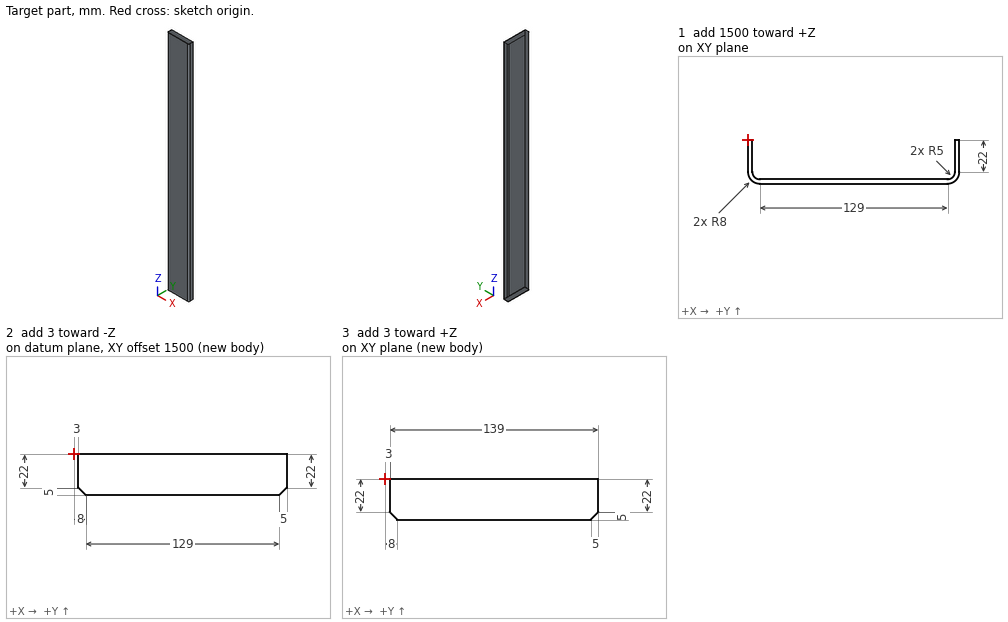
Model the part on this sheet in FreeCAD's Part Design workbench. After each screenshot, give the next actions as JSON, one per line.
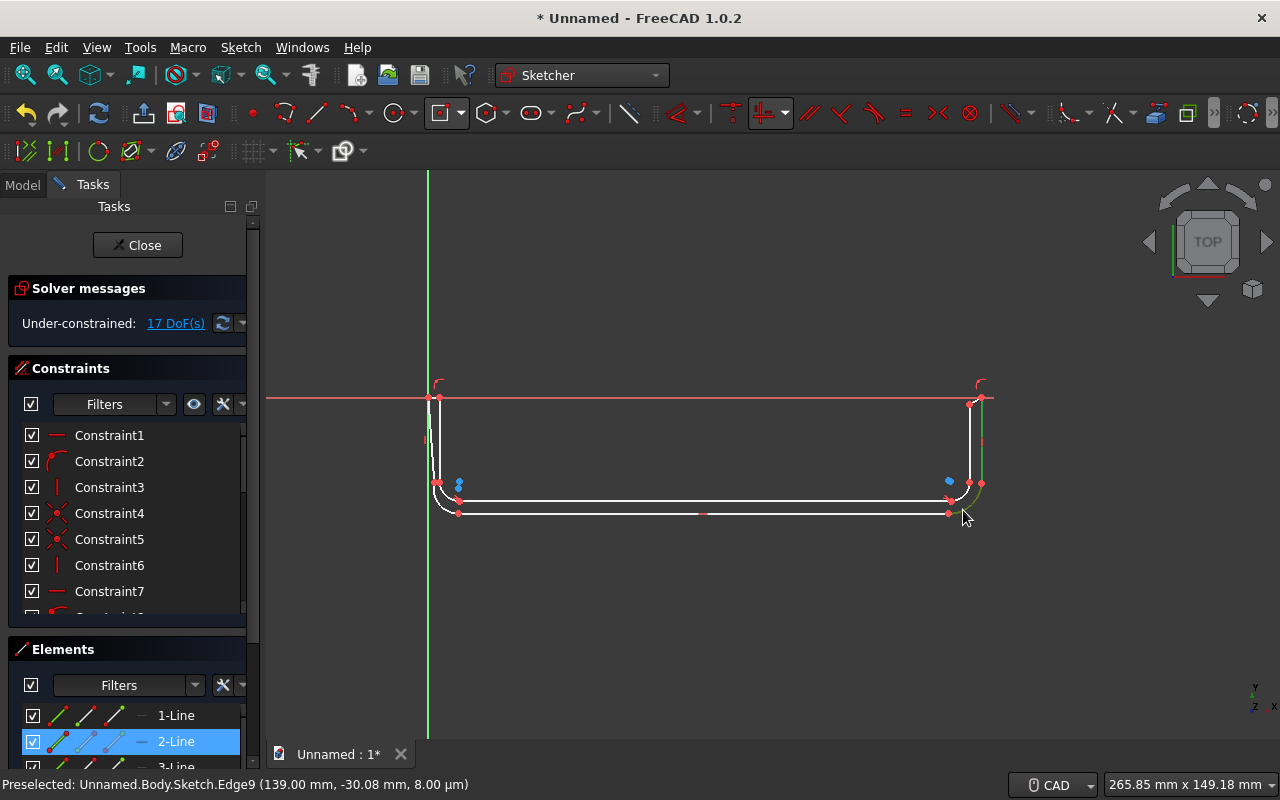
{"action": "key", "text": "t"}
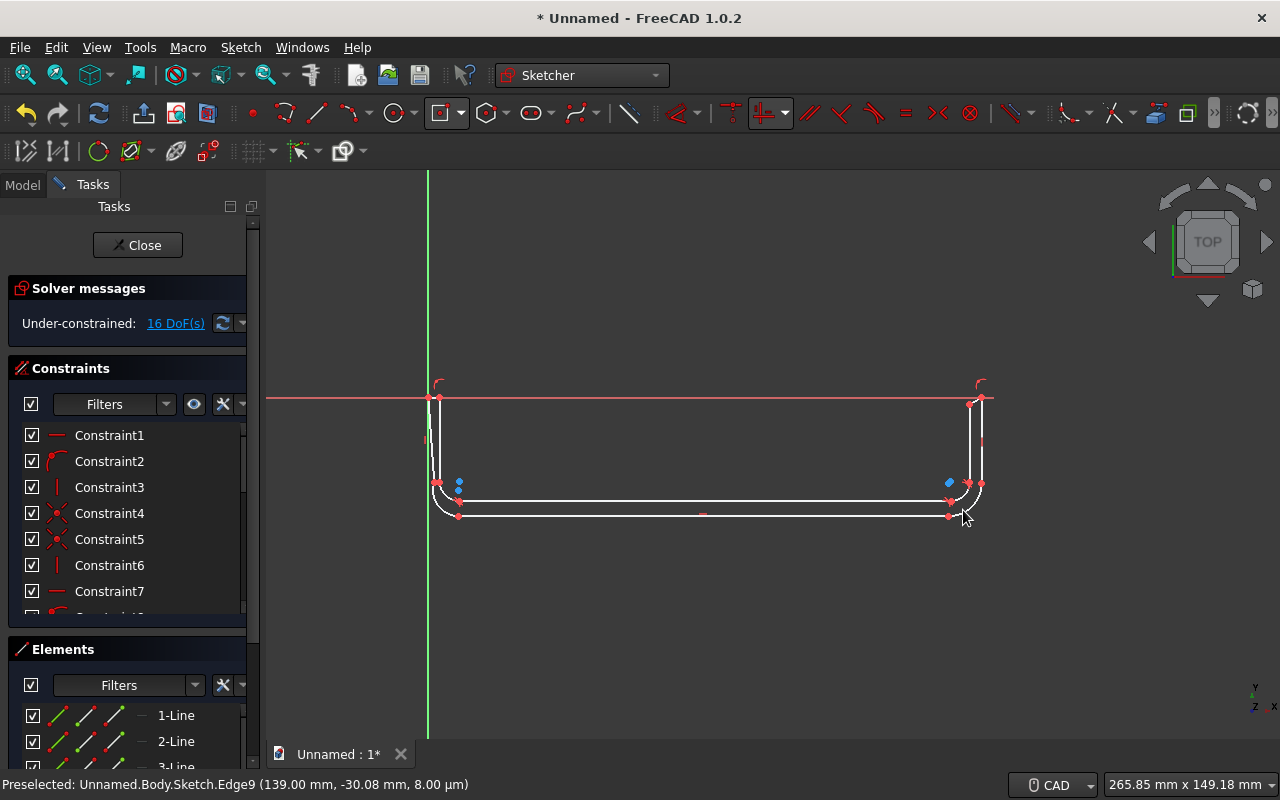
{"action": "left_click", "coordinate": [970, 428]}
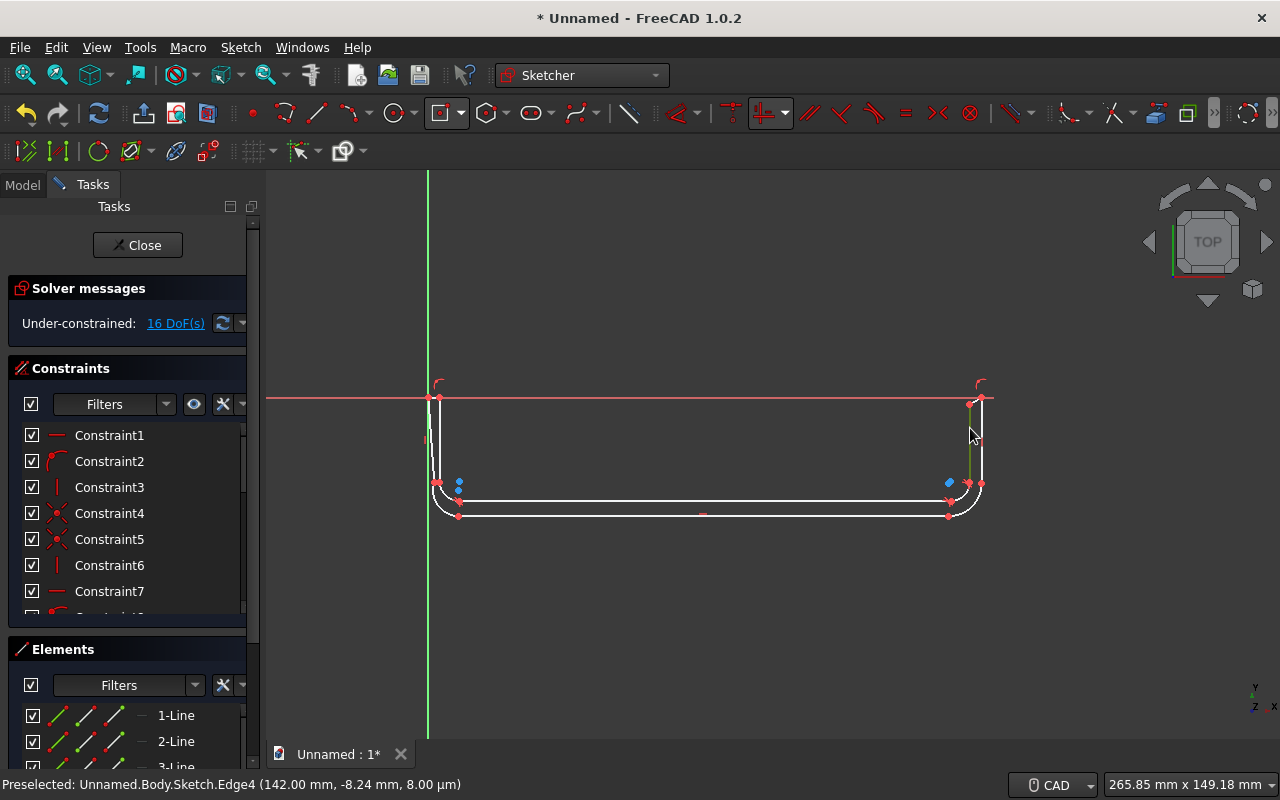
{"action": "left_click", "coordinate": [964, 495]}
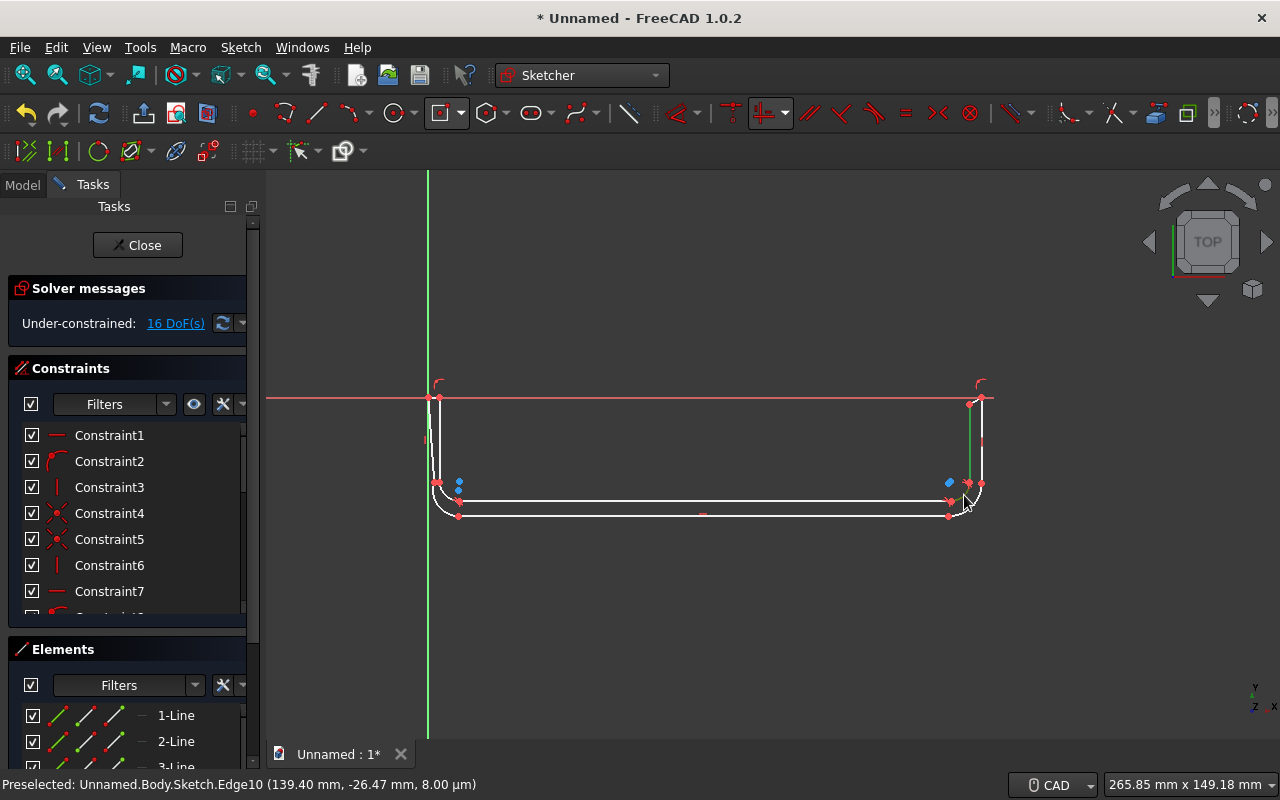
{"action": "key", "text": "t"}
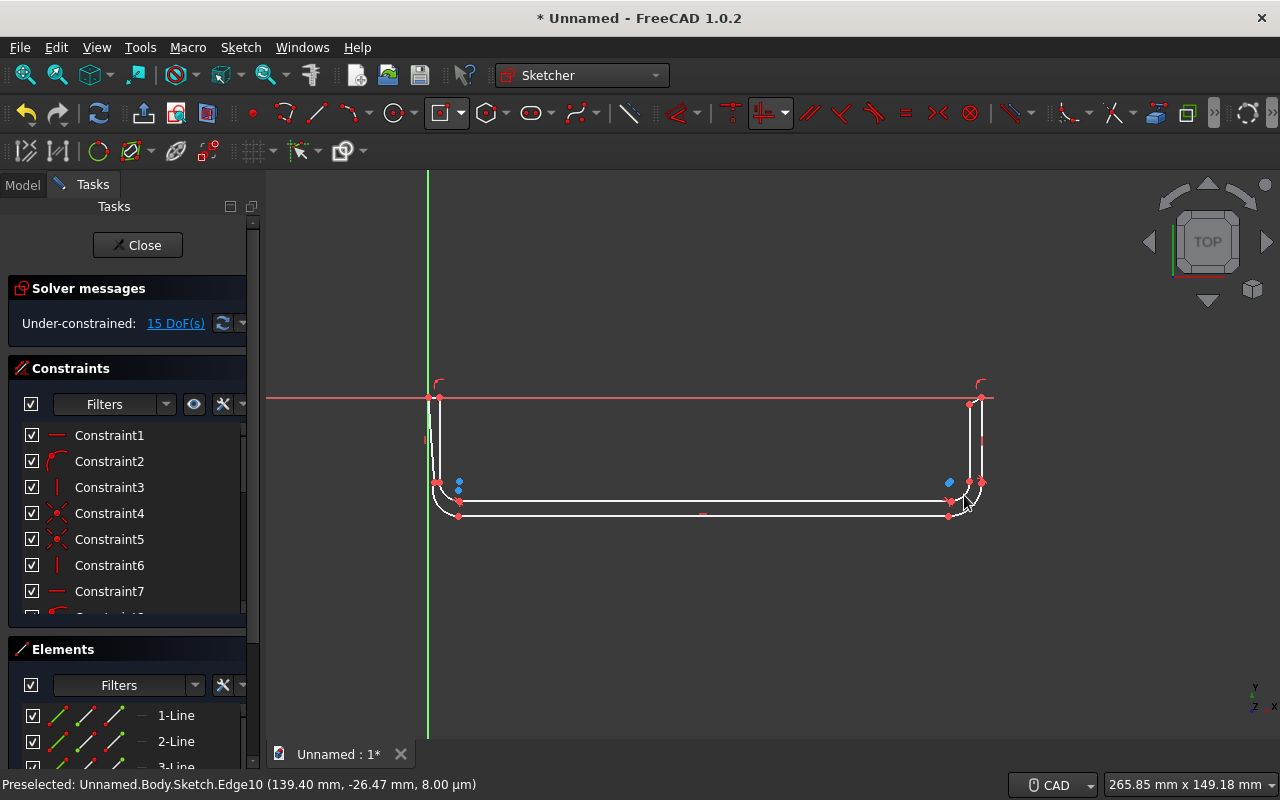
{"action": "left_click", "coordinate": [804, 501]}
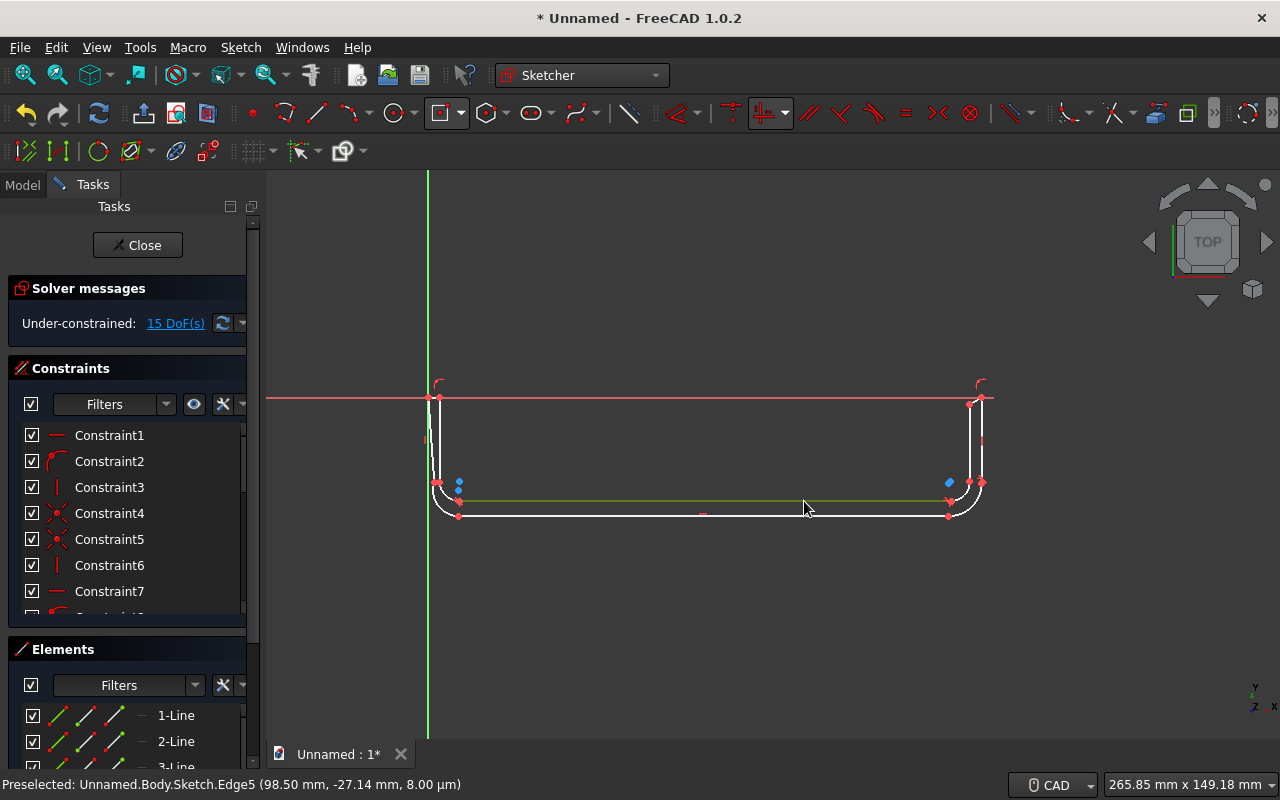
{"action": "left_click", "coordinate": [964, 495]}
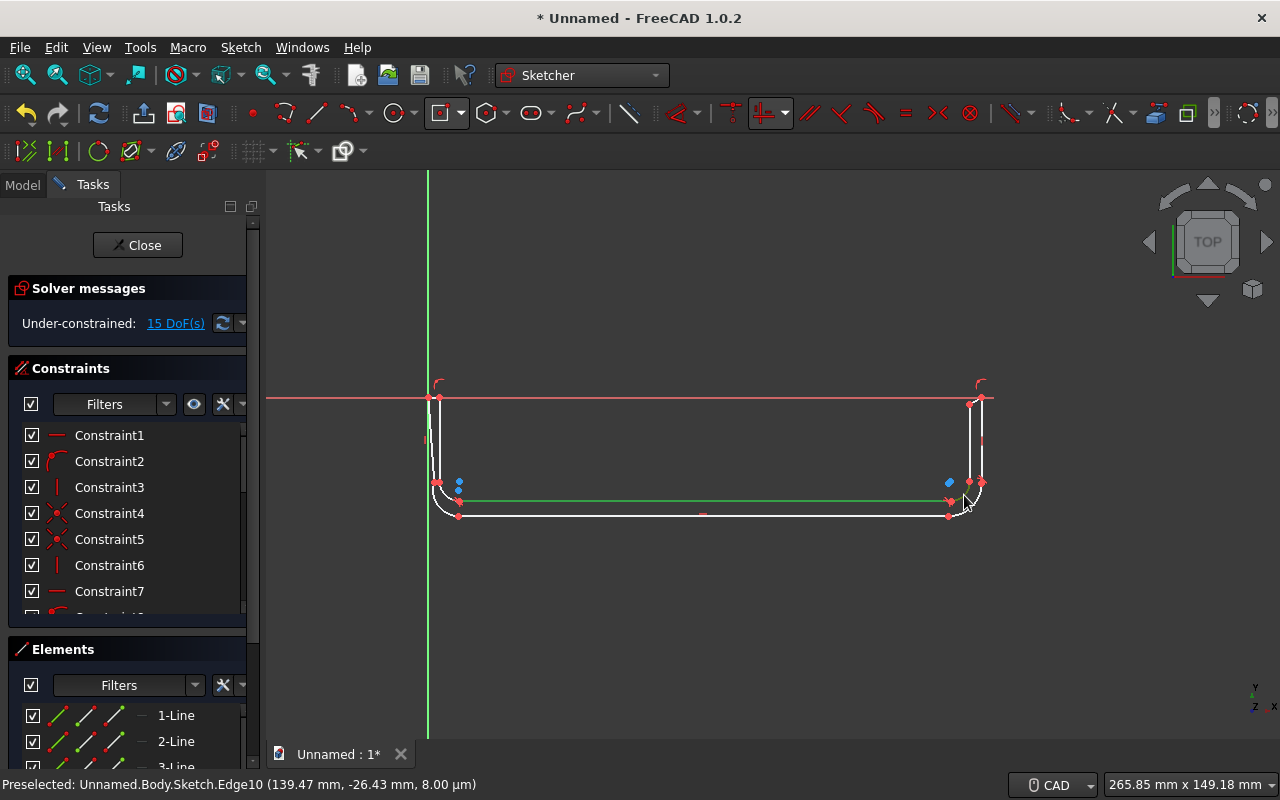
{"action": "key", "text": "t"}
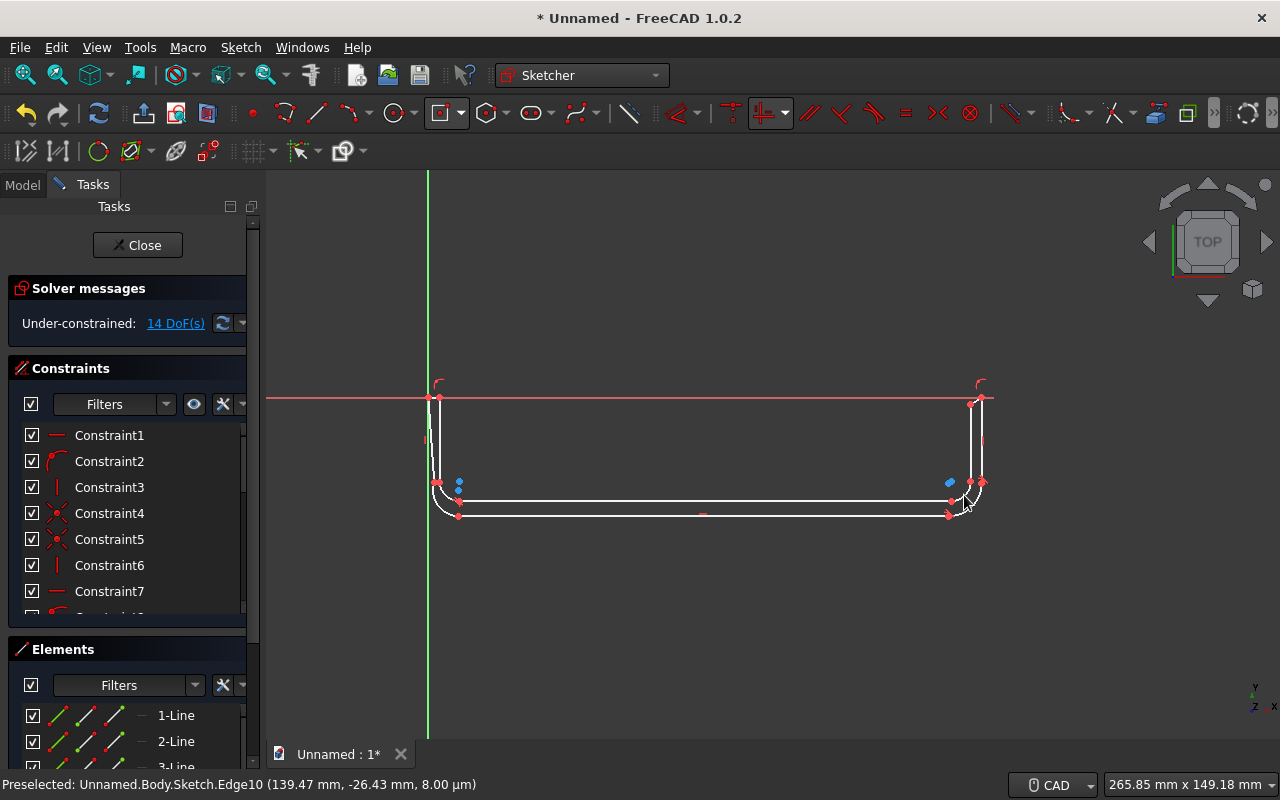
{"action": "left_click", "coordinate": [804, 501]}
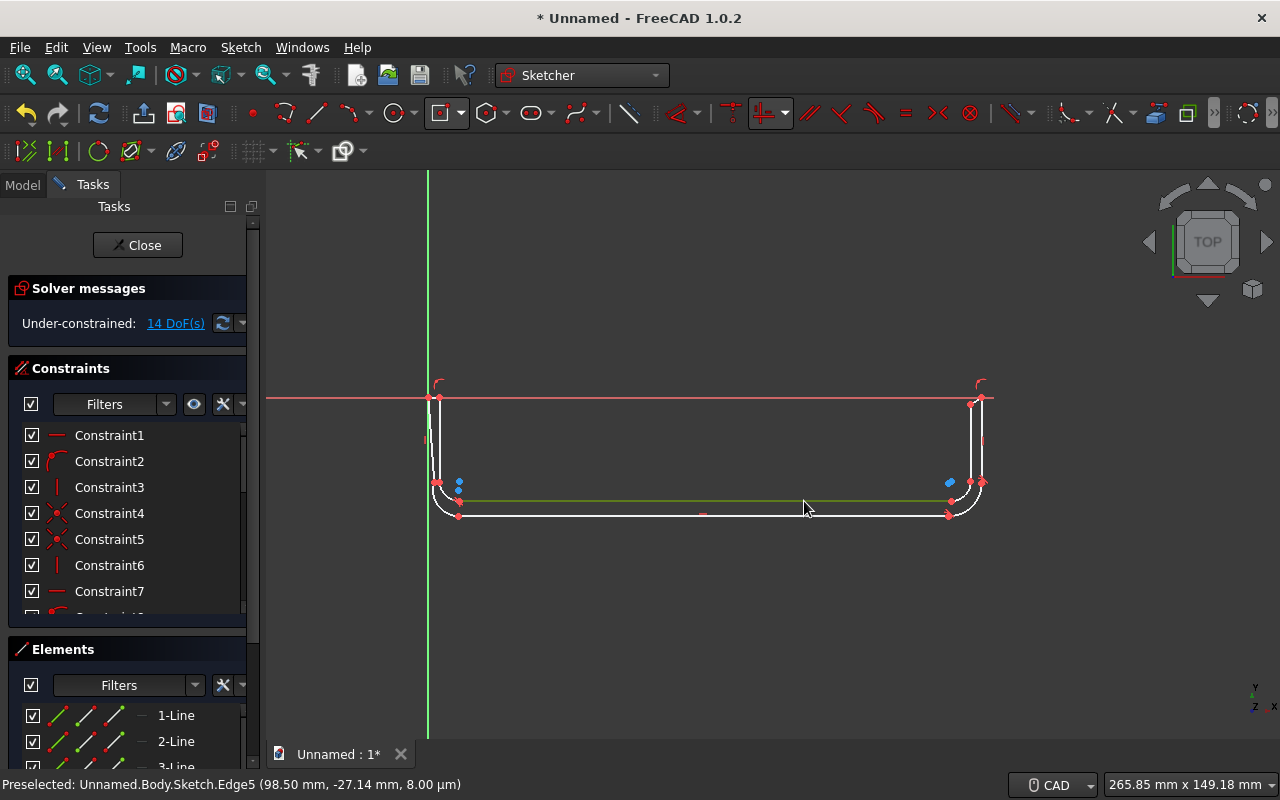
{"action": "left_click", "coordinate": [446, 496]}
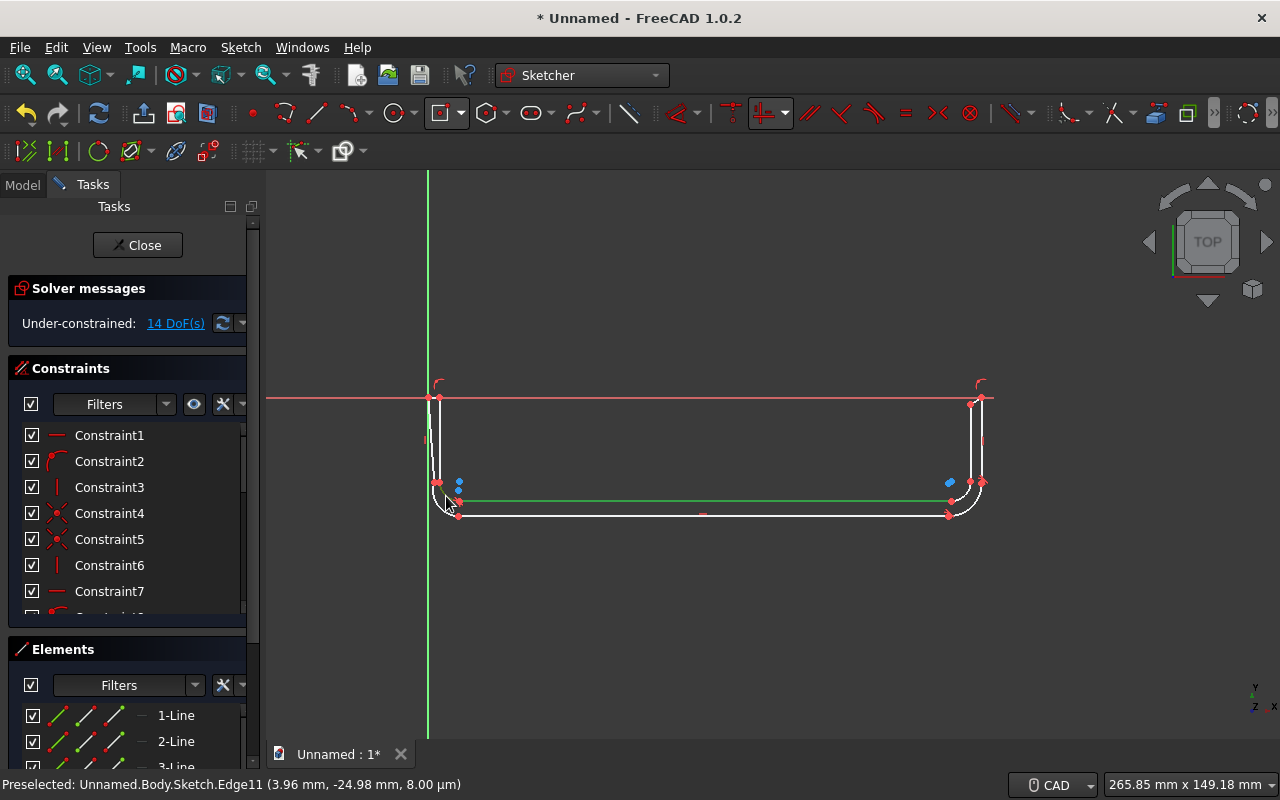
{"action": "key", "text": "t"}